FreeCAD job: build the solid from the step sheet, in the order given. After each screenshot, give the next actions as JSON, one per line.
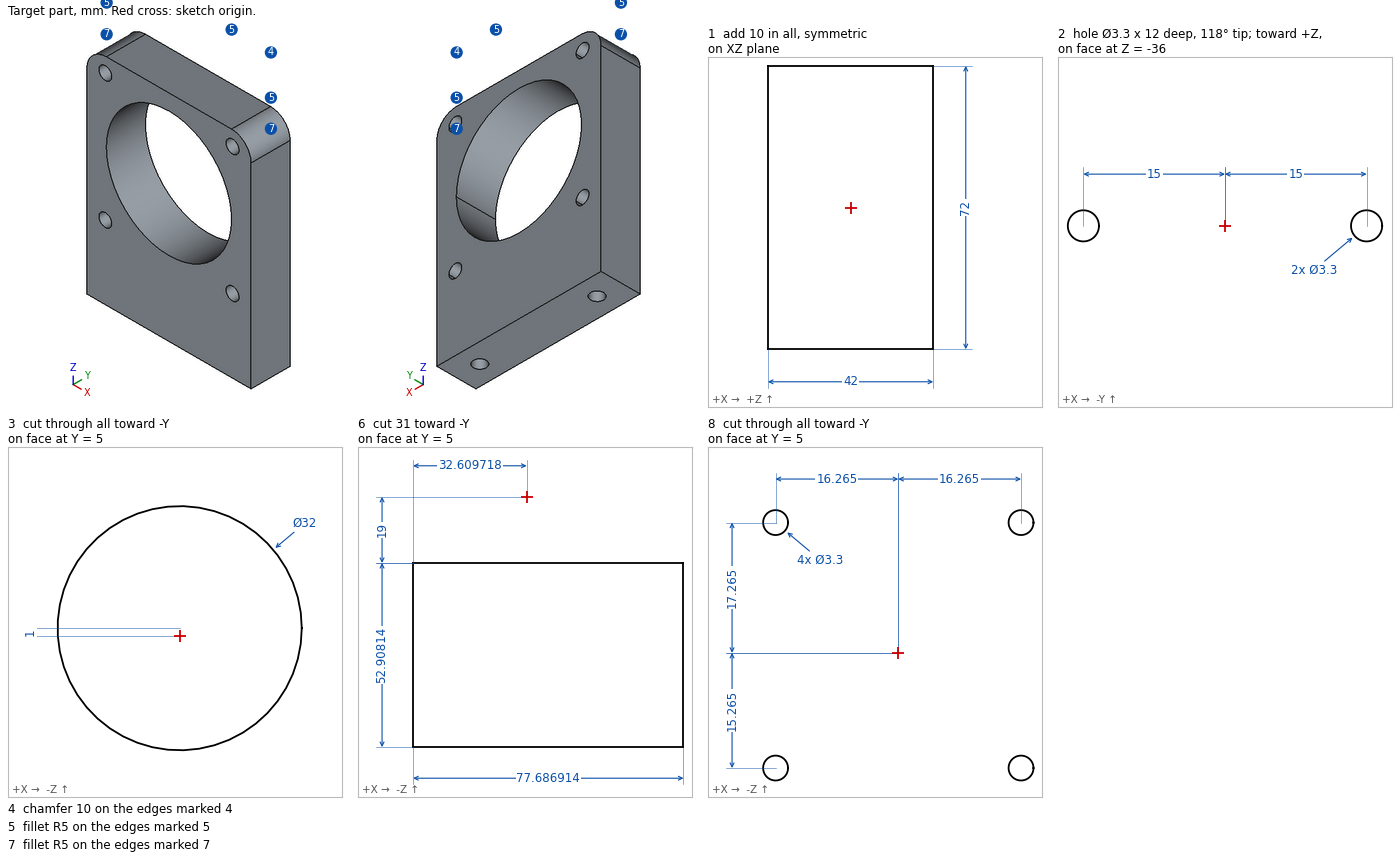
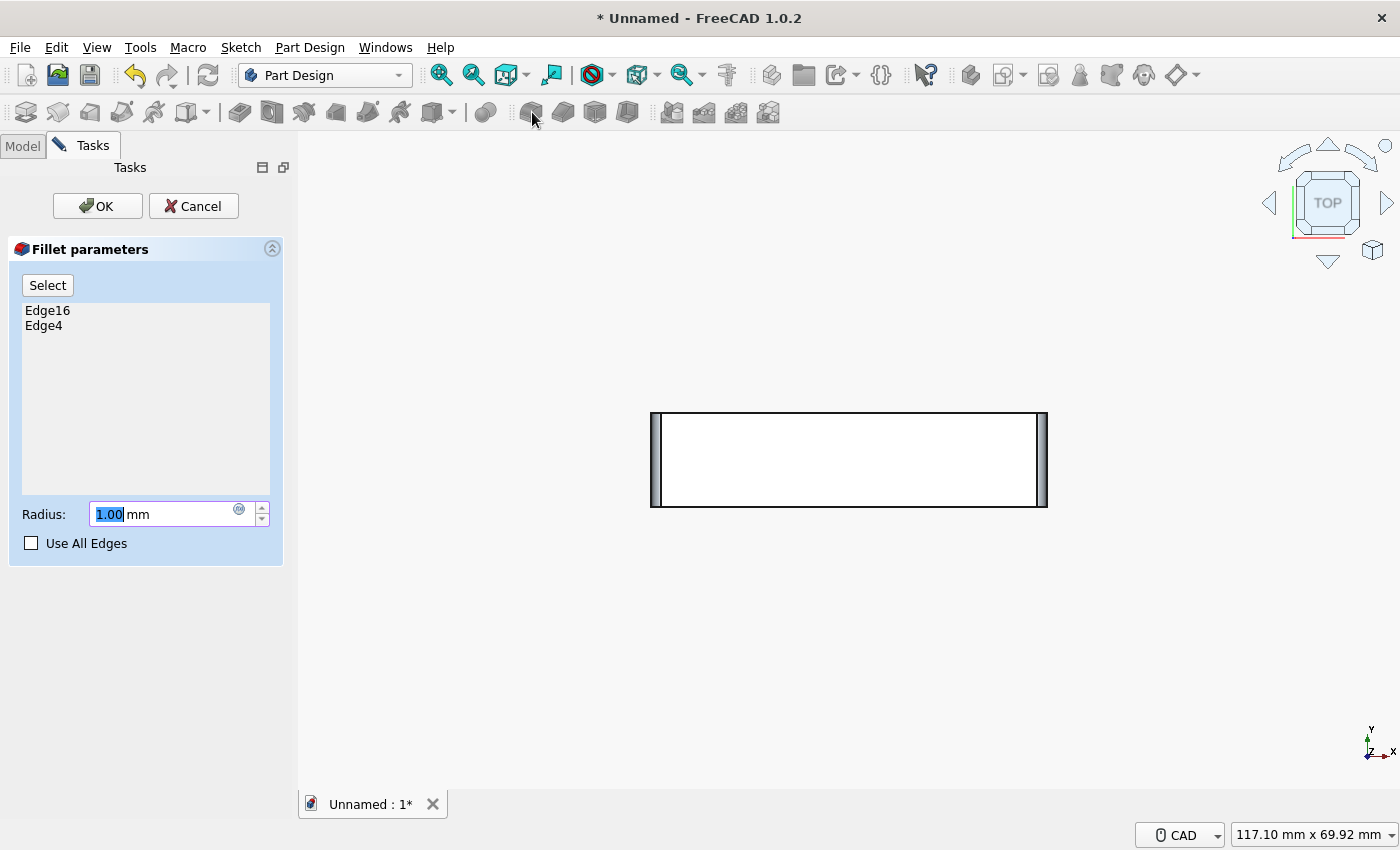
{"action": "type", "text": "5"}
{"action": "key", "text": "Tab"}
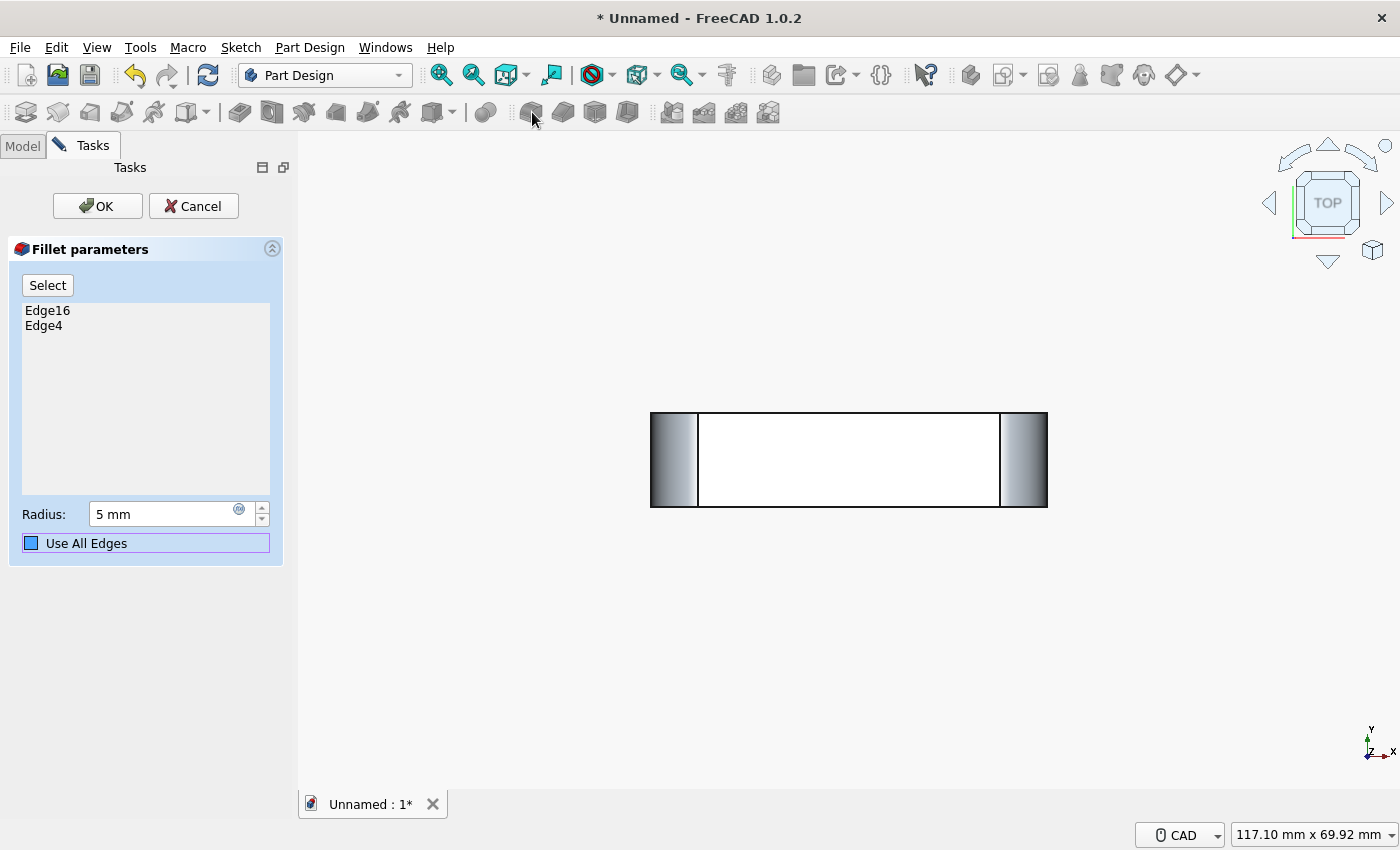
{"action": "left_click", "coordinate": [98, 206]}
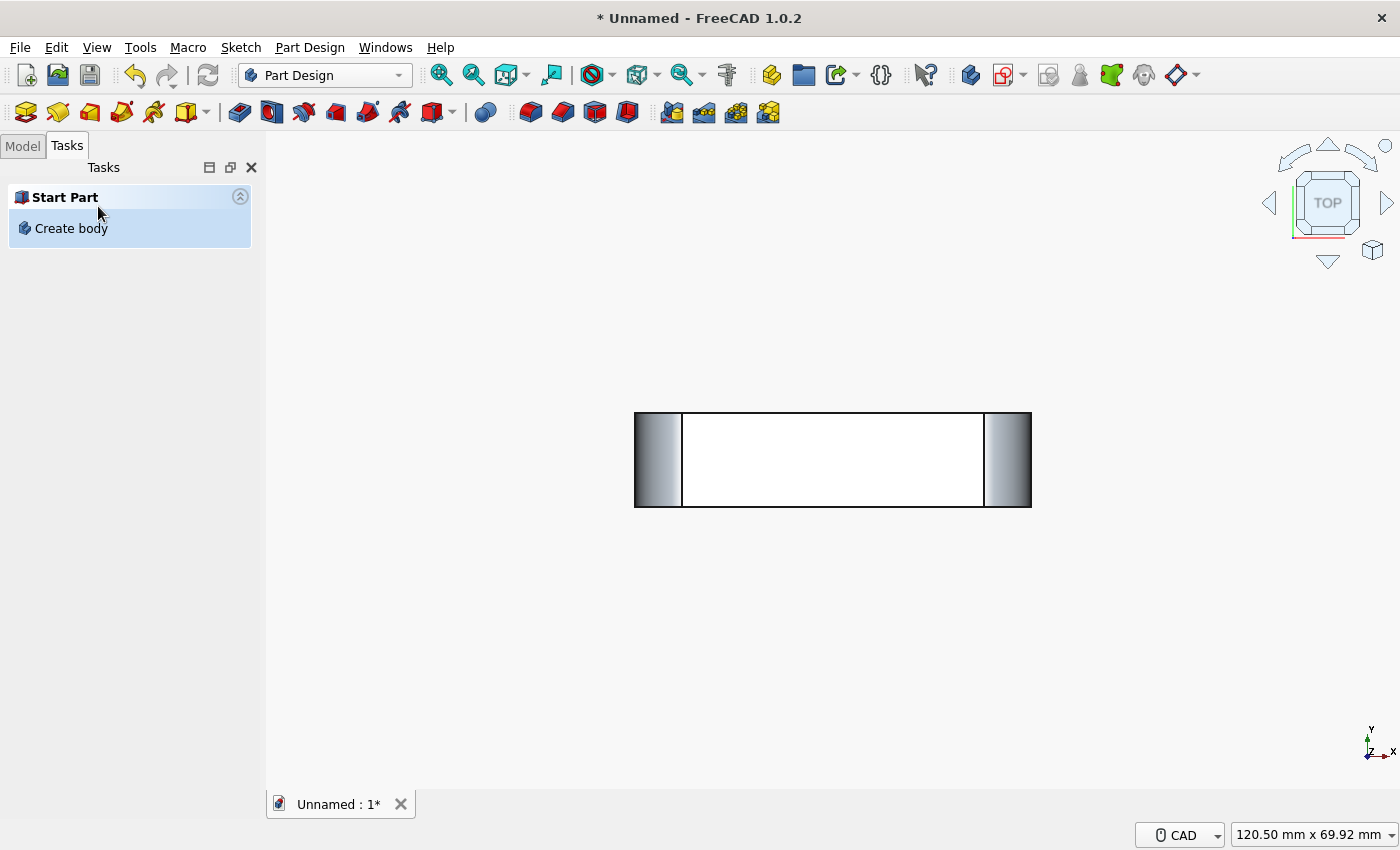
{"action": "key", "text": "v f"}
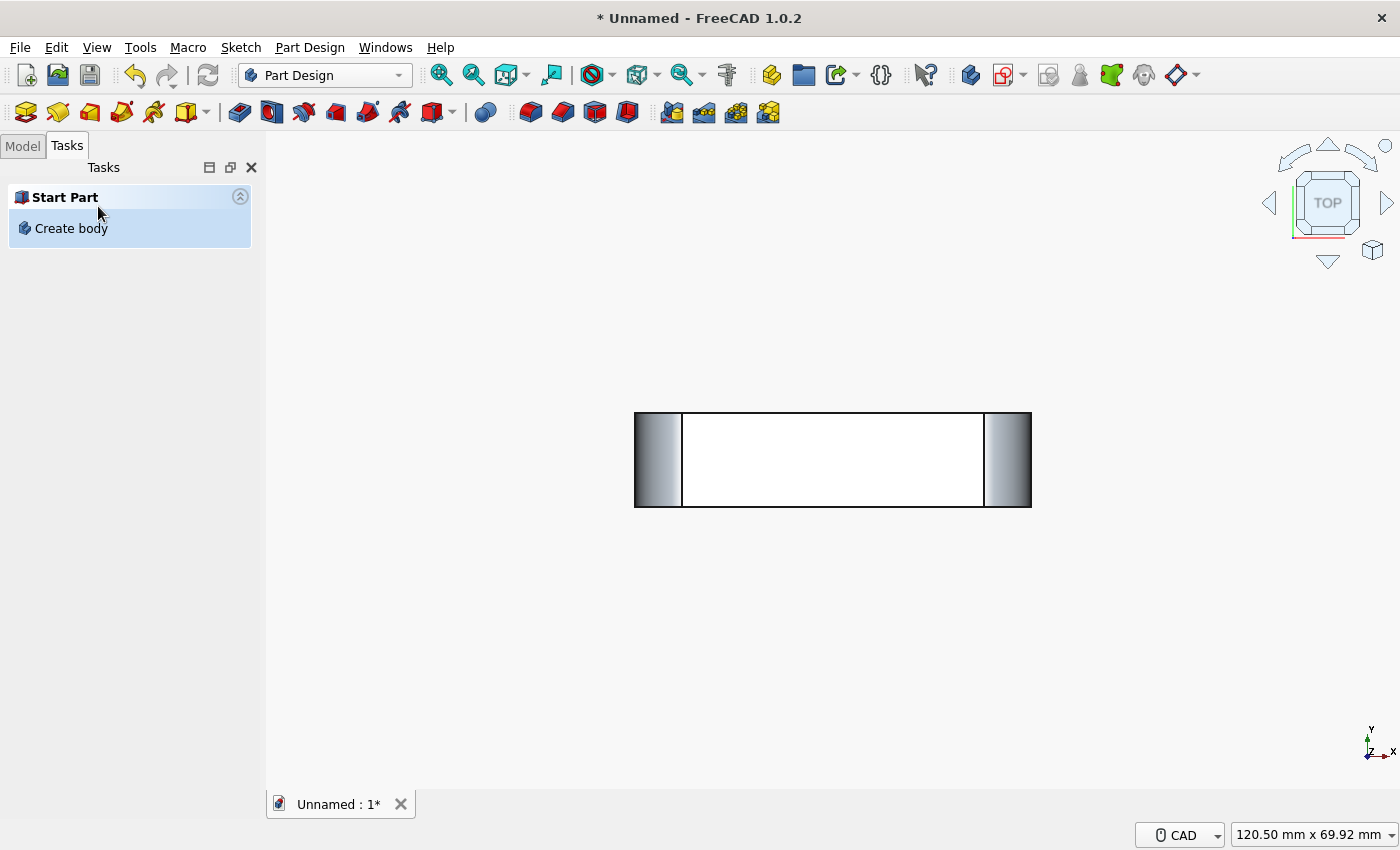
{"action": "key", "text": "4"}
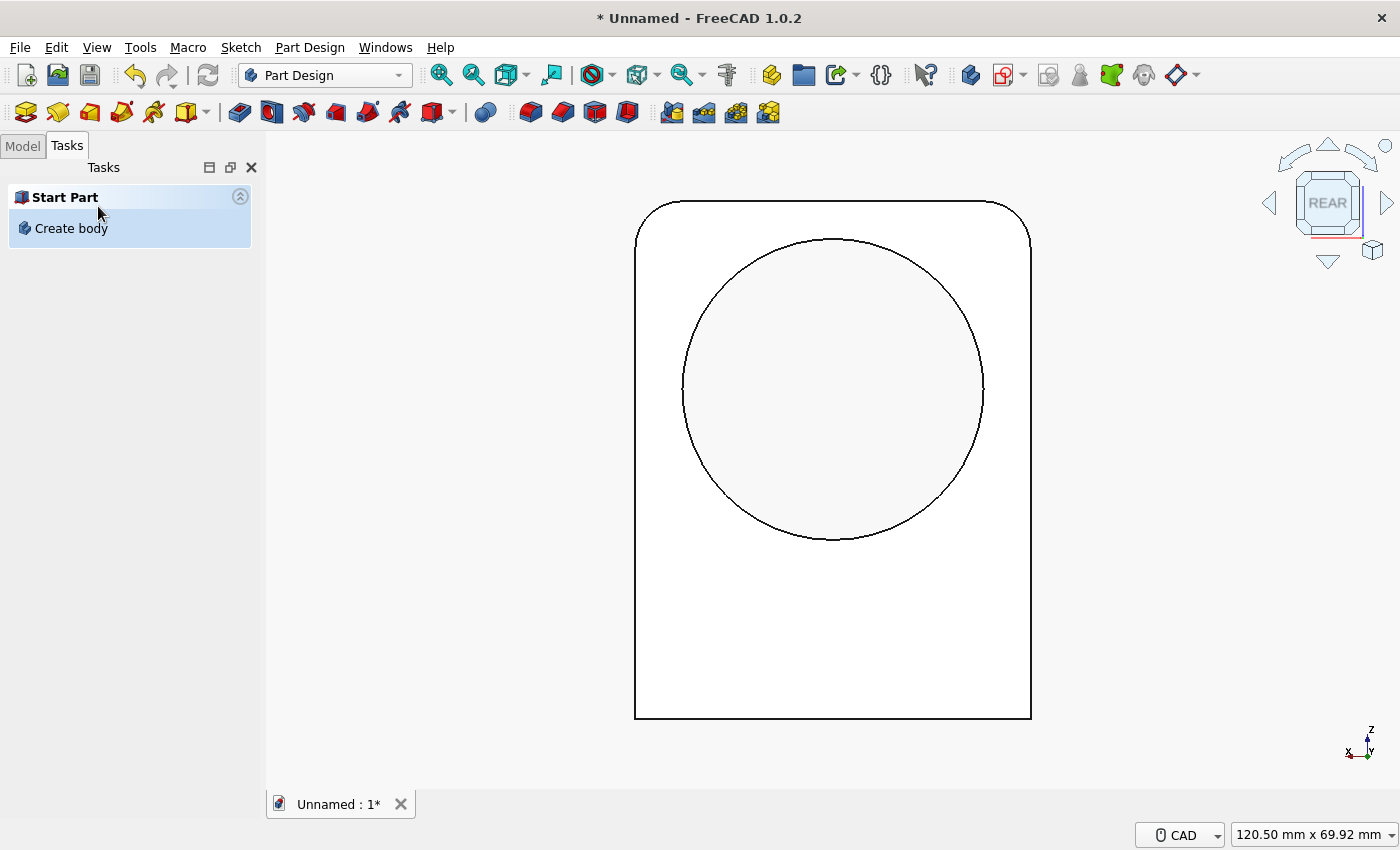
{"action": "left_click", "coordinate": [720, 607]}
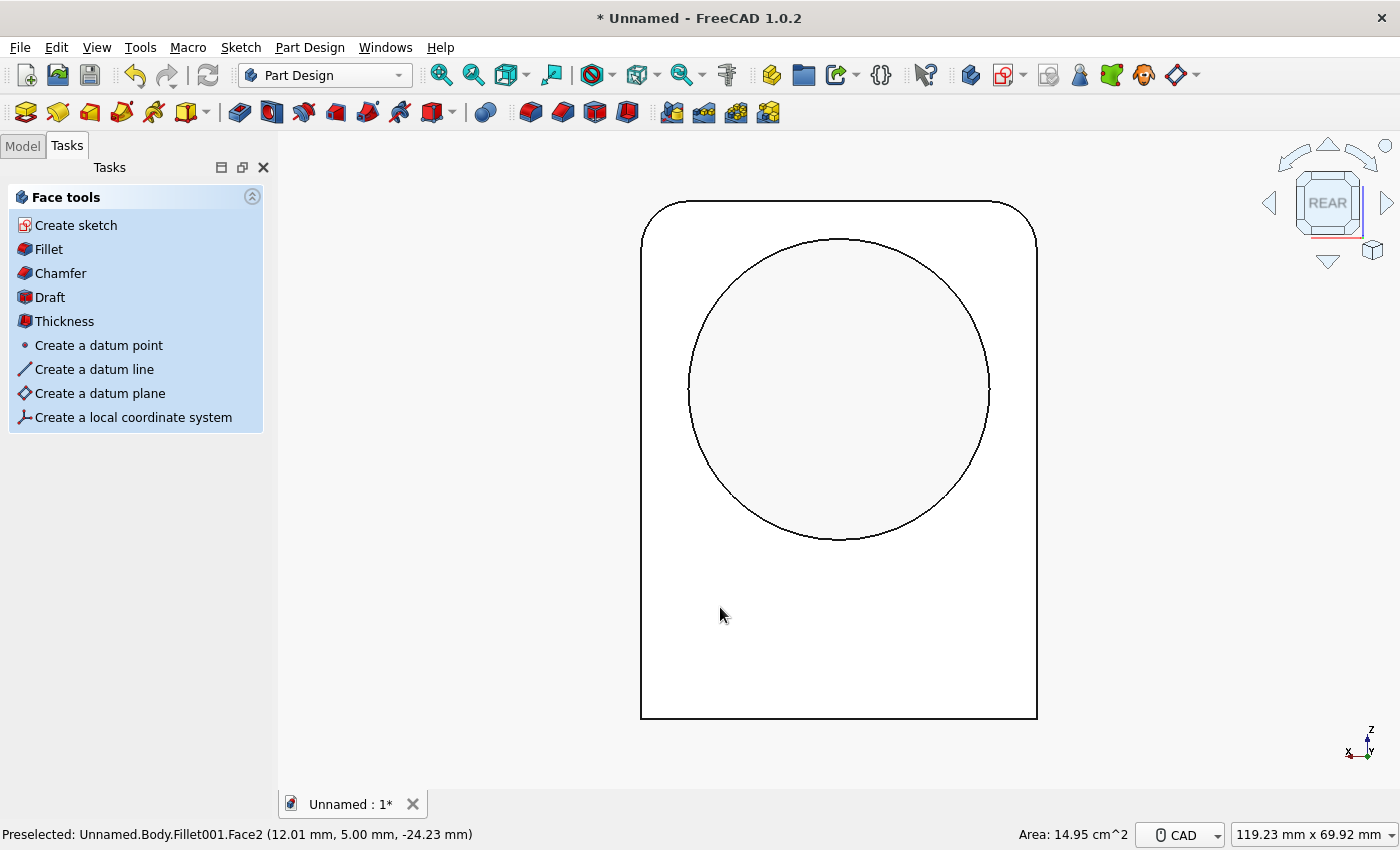
{"action": "left_click", "coordinate": [1004, 76]}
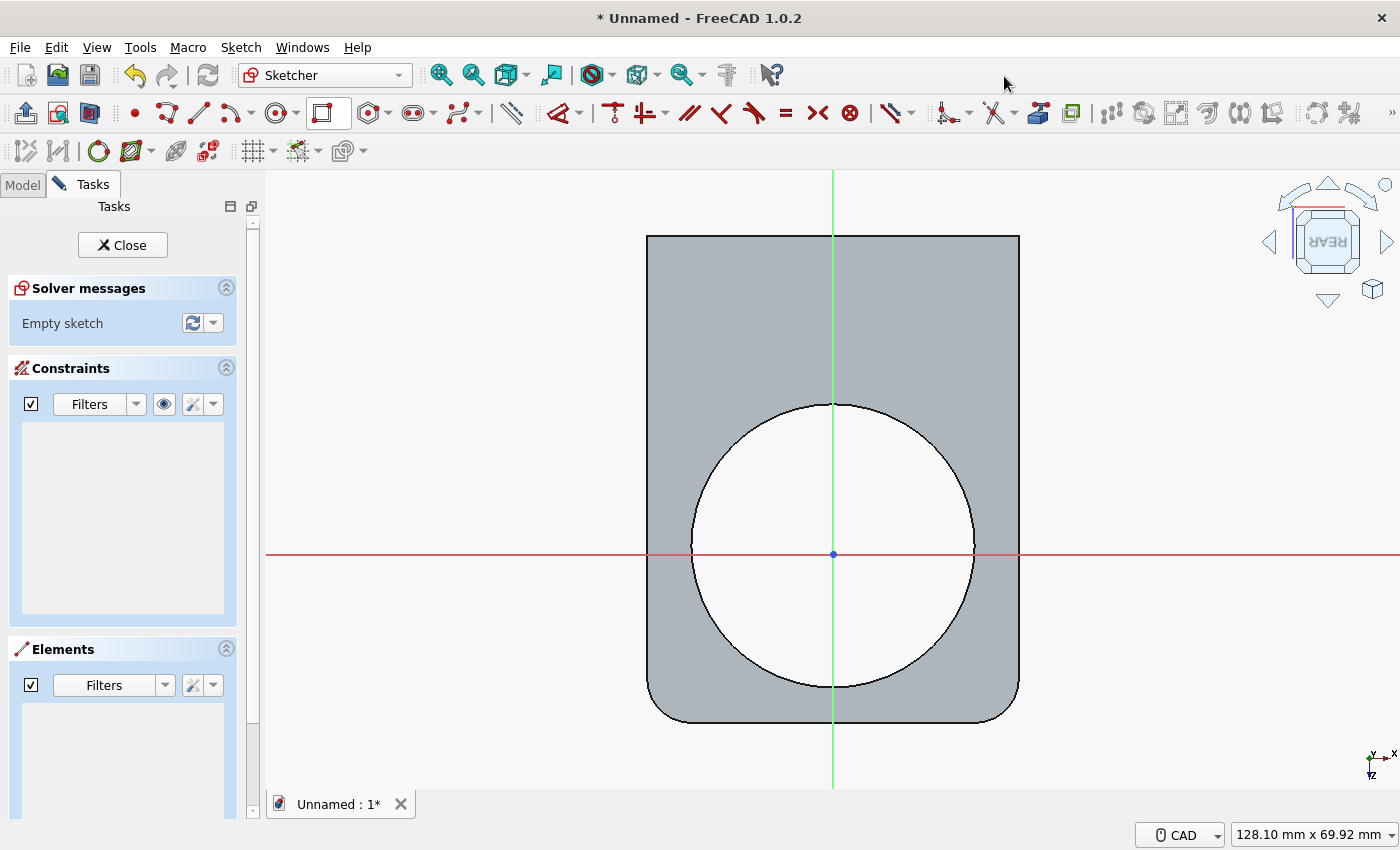
{"action": "key", "text": "g c"}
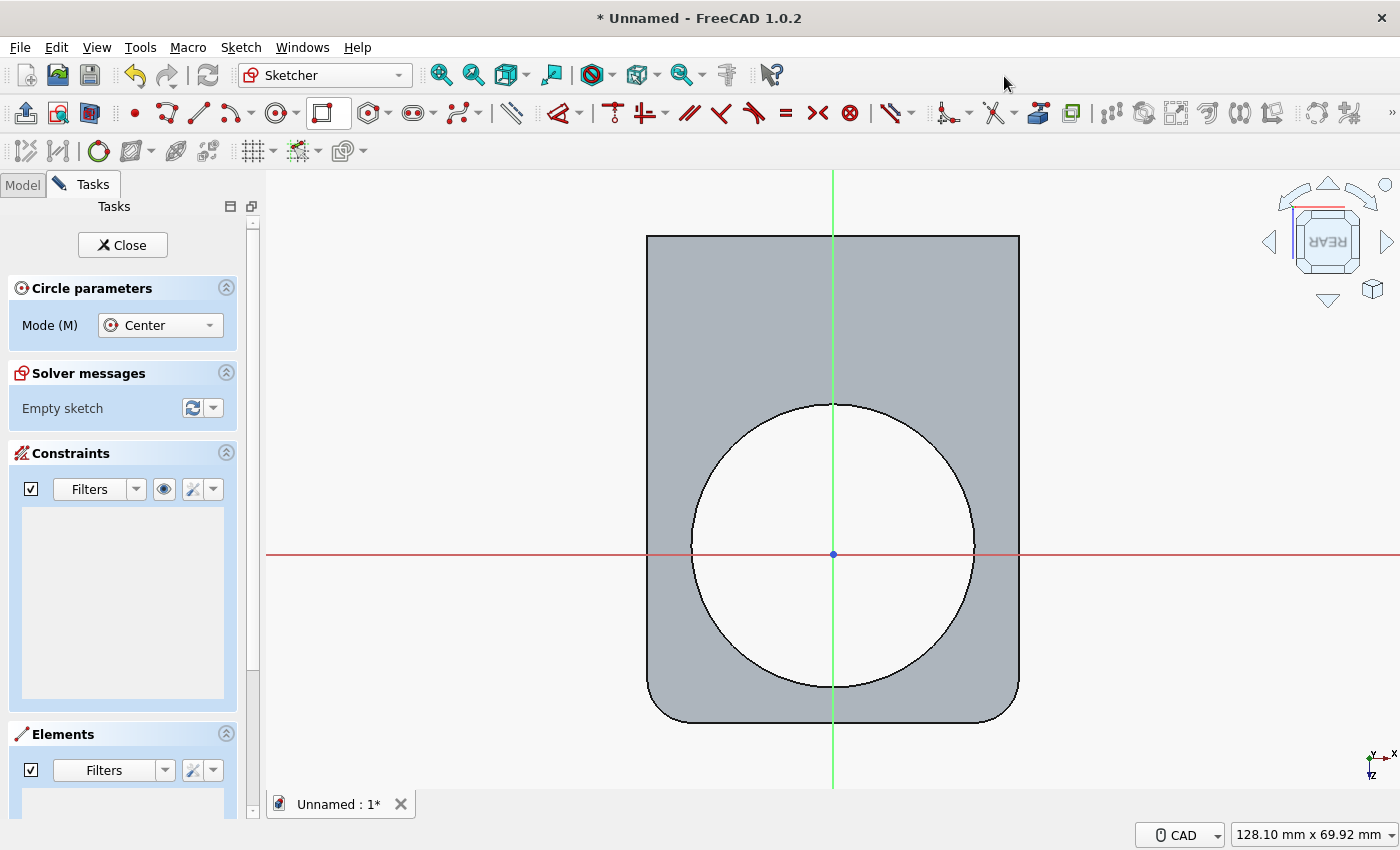
{"action": "scroll", "coordinate": [689, 402], "scroll_direction": "up", "scroll_amount": 3}